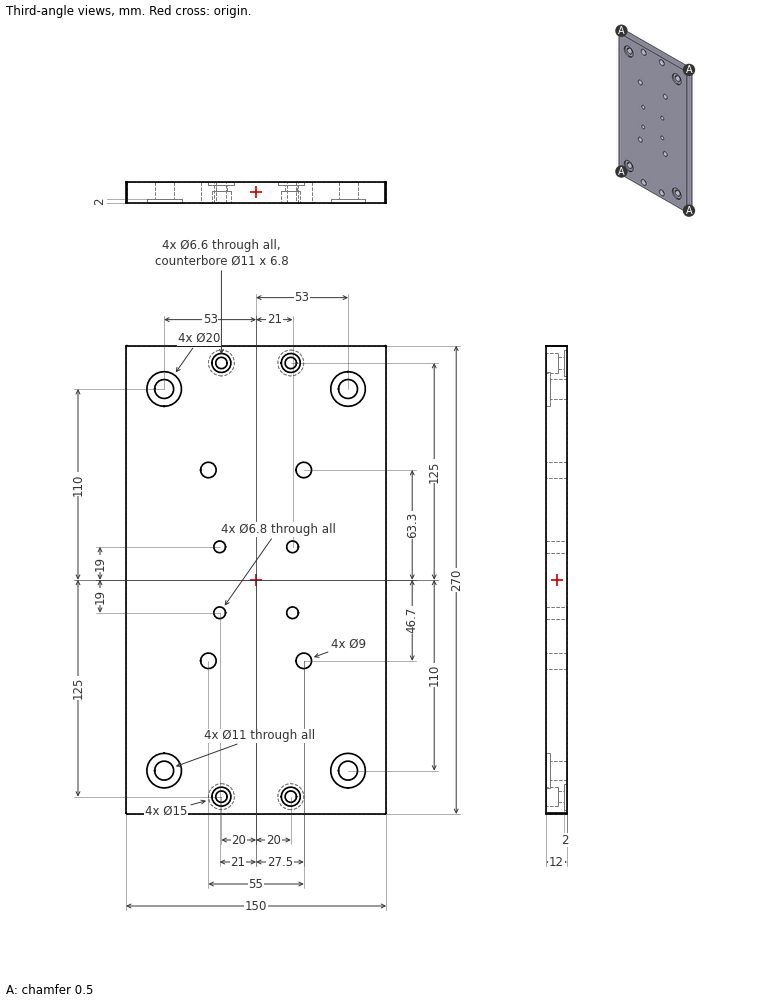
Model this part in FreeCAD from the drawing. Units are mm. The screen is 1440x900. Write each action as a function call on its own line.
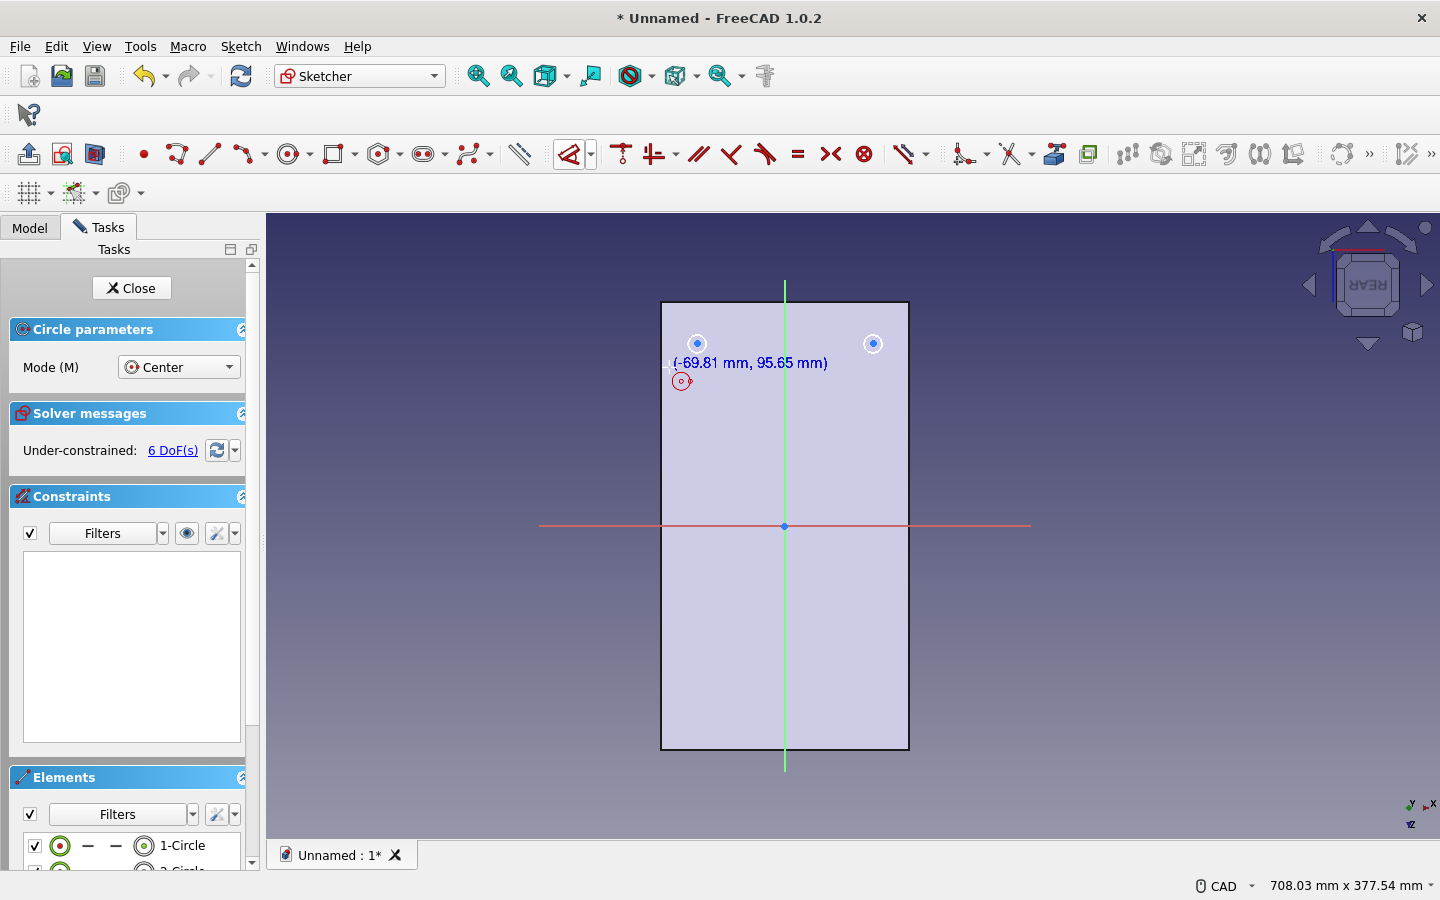
scroll(697, 709, up, 5)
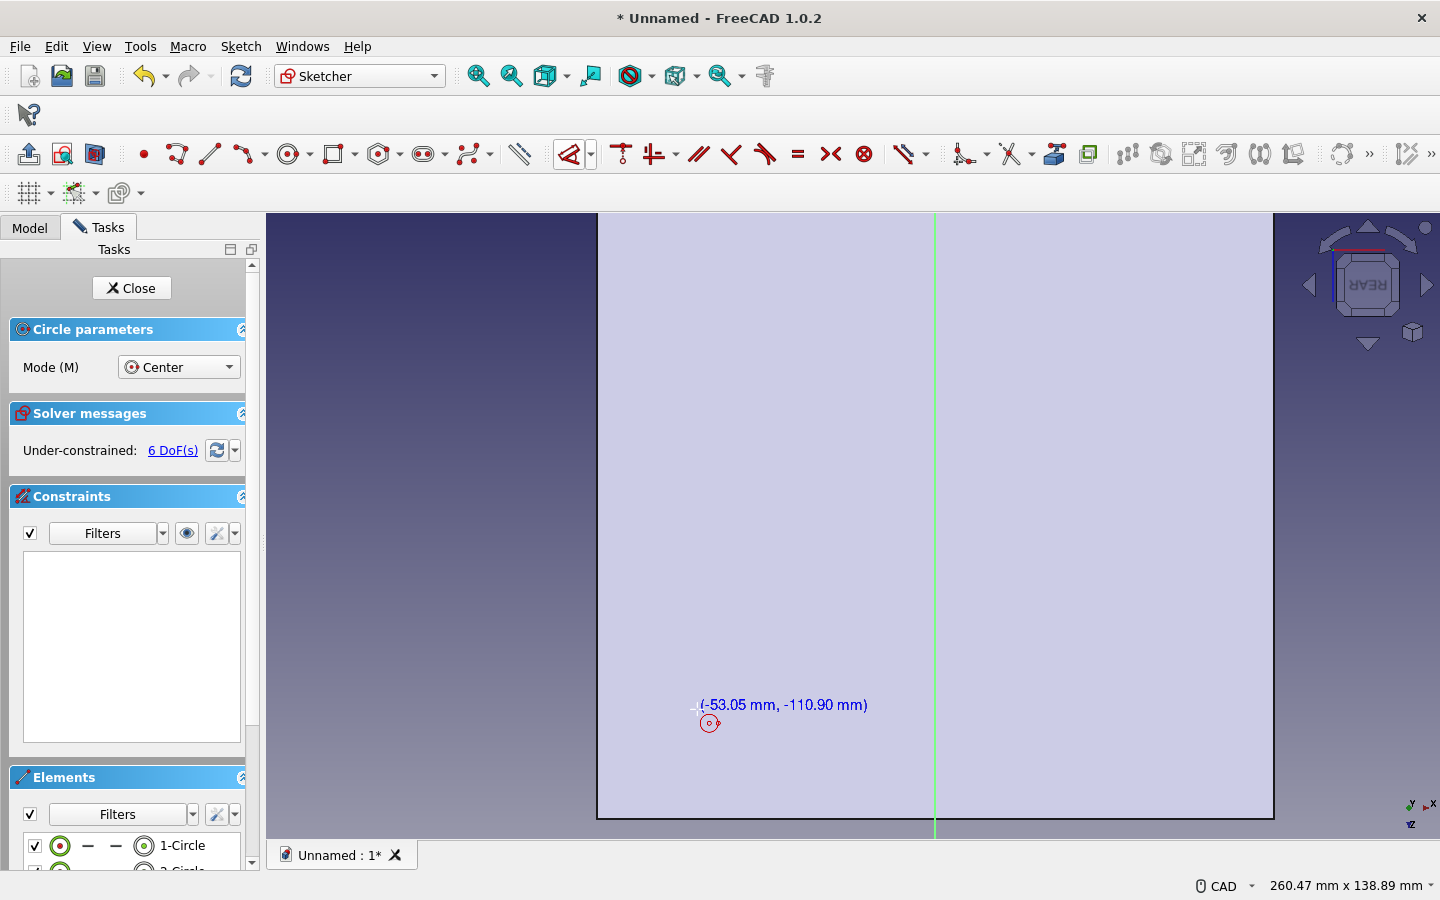
click(697, 706)
click(714, 689)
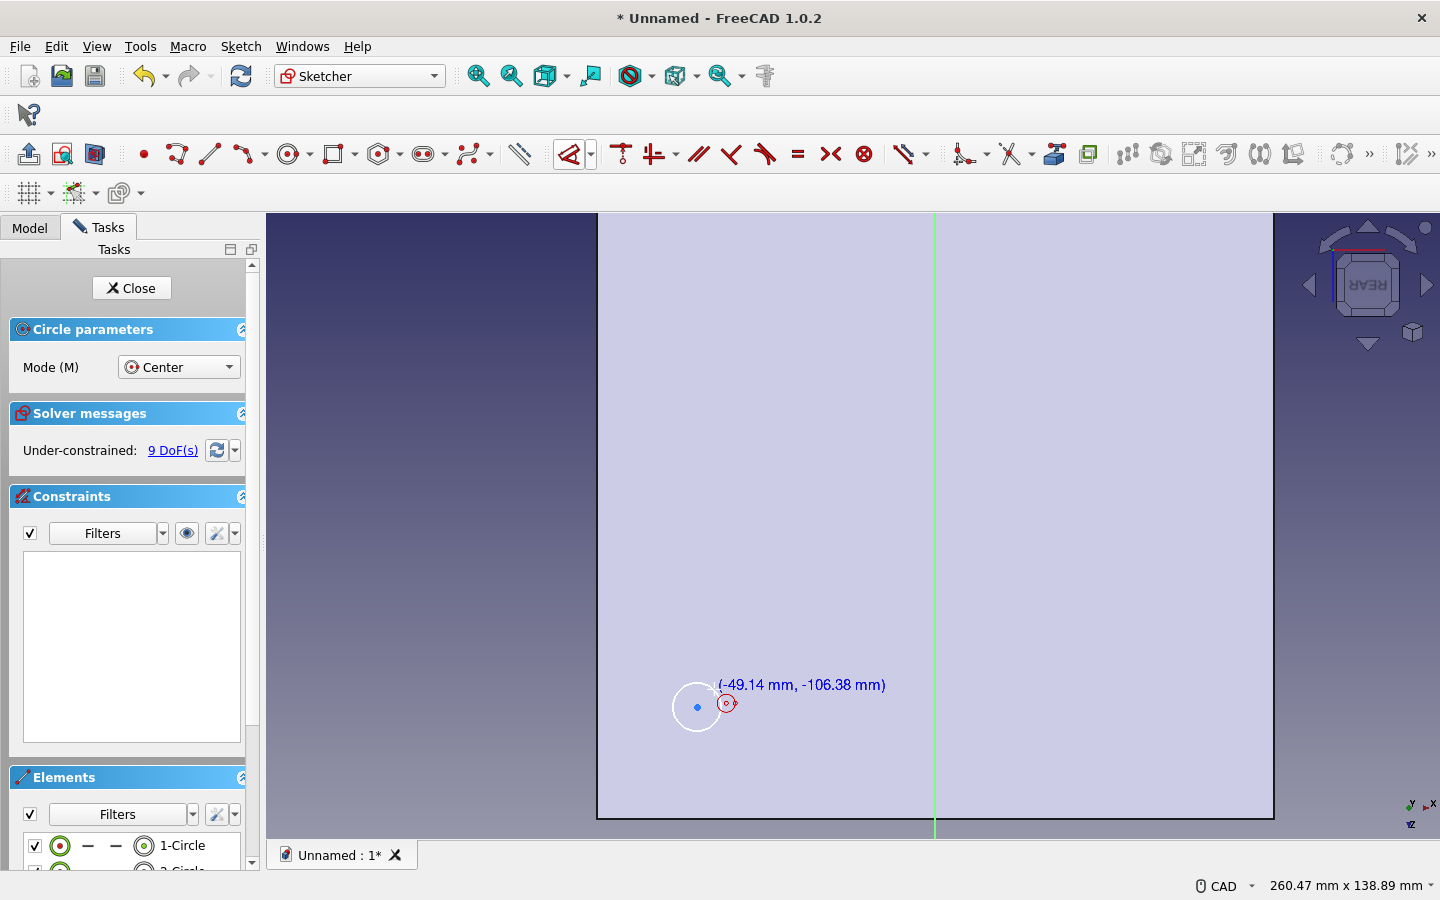
click(1174, 706)
click(1192, 689)
key(Escape)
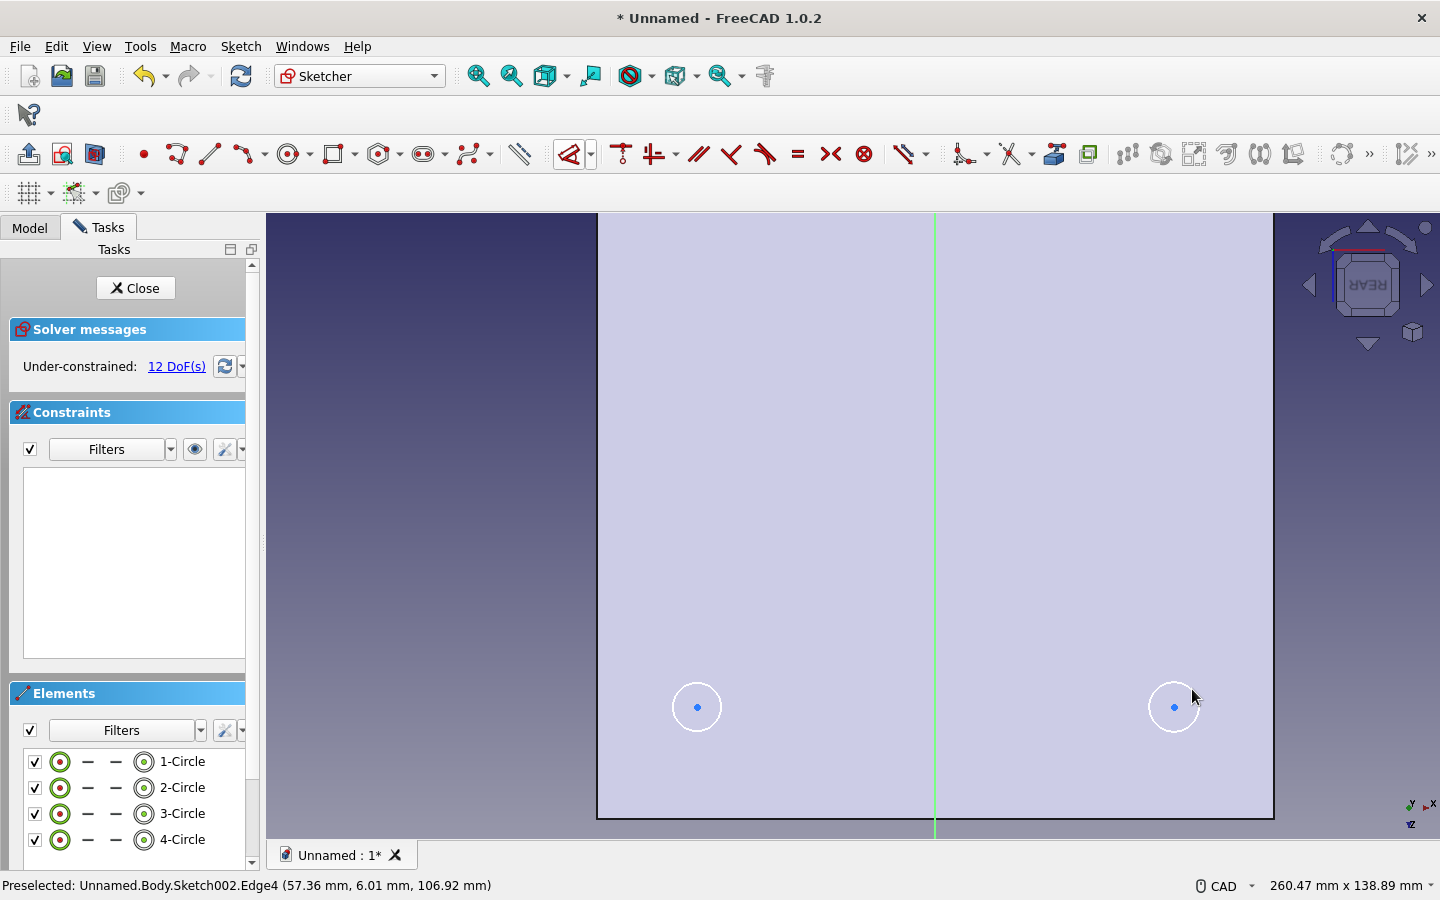
scroll(697, 710, down, 5)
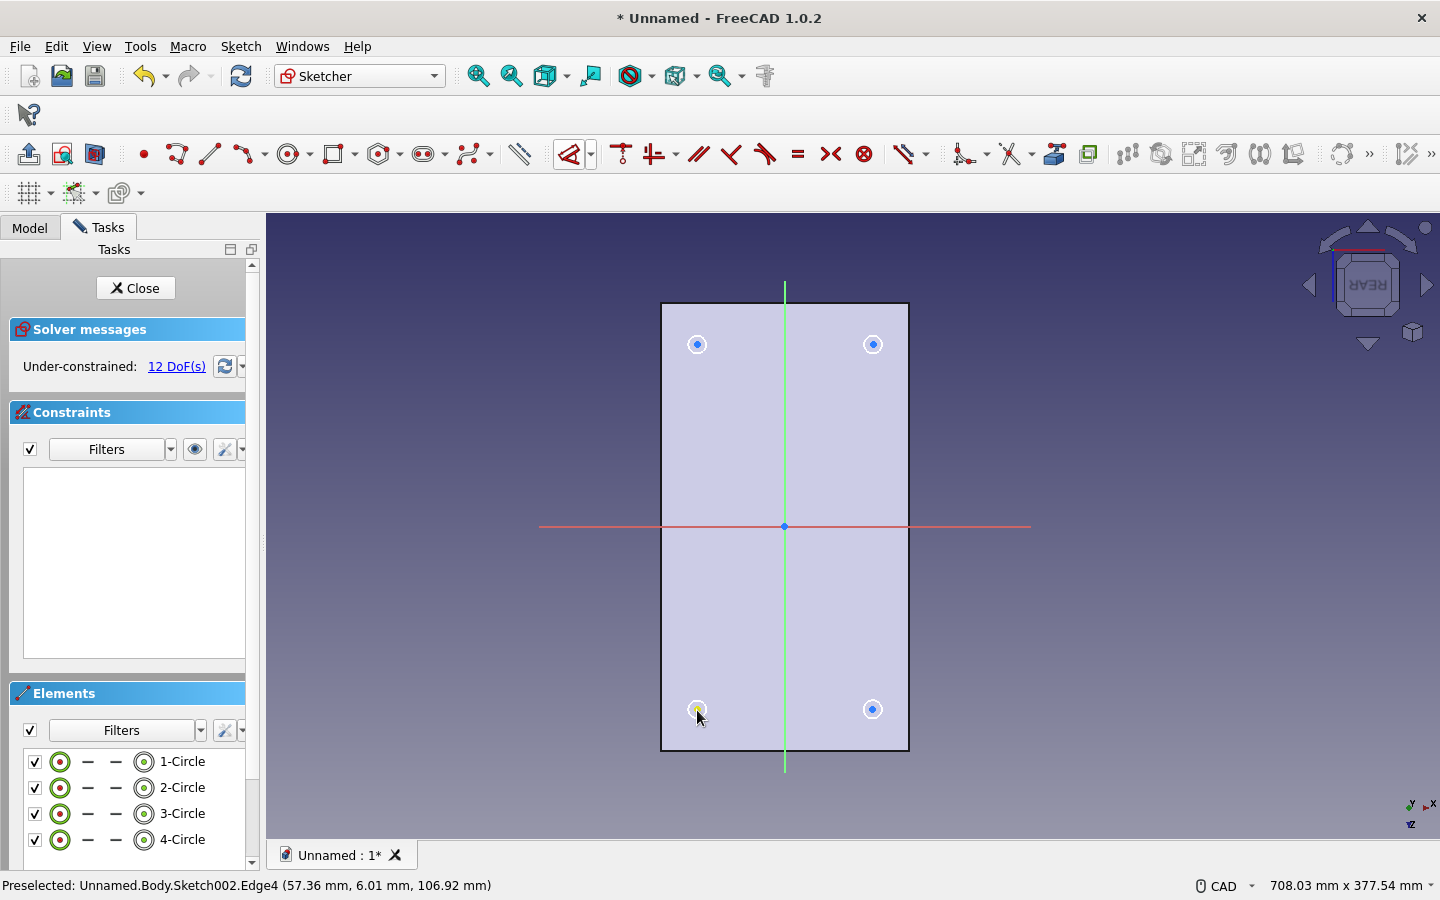
scroll(703, 338, up, 3)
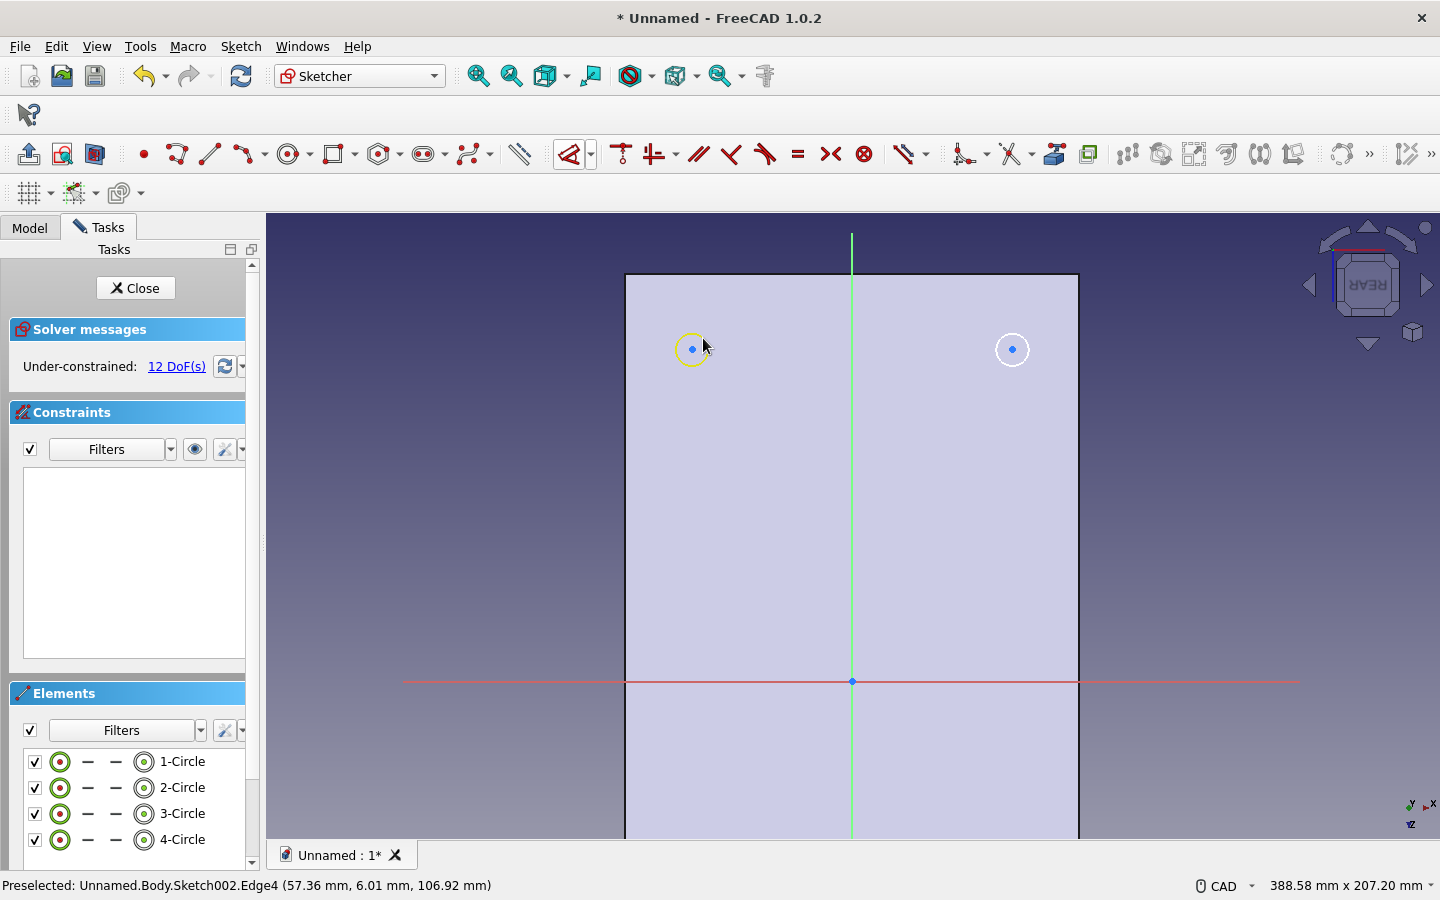
click(703, 338)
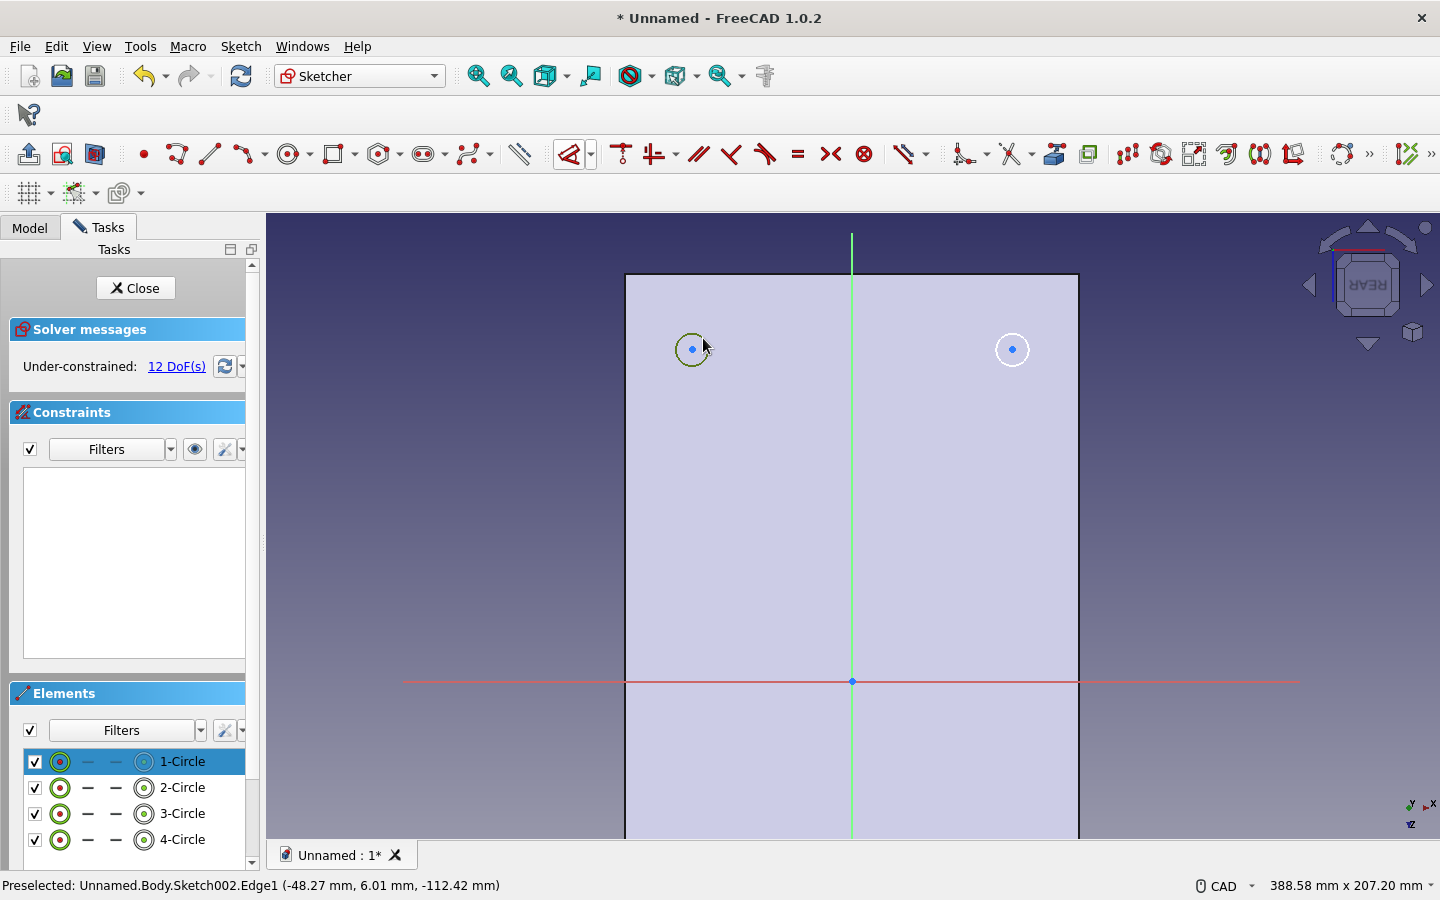
click(1024, 338)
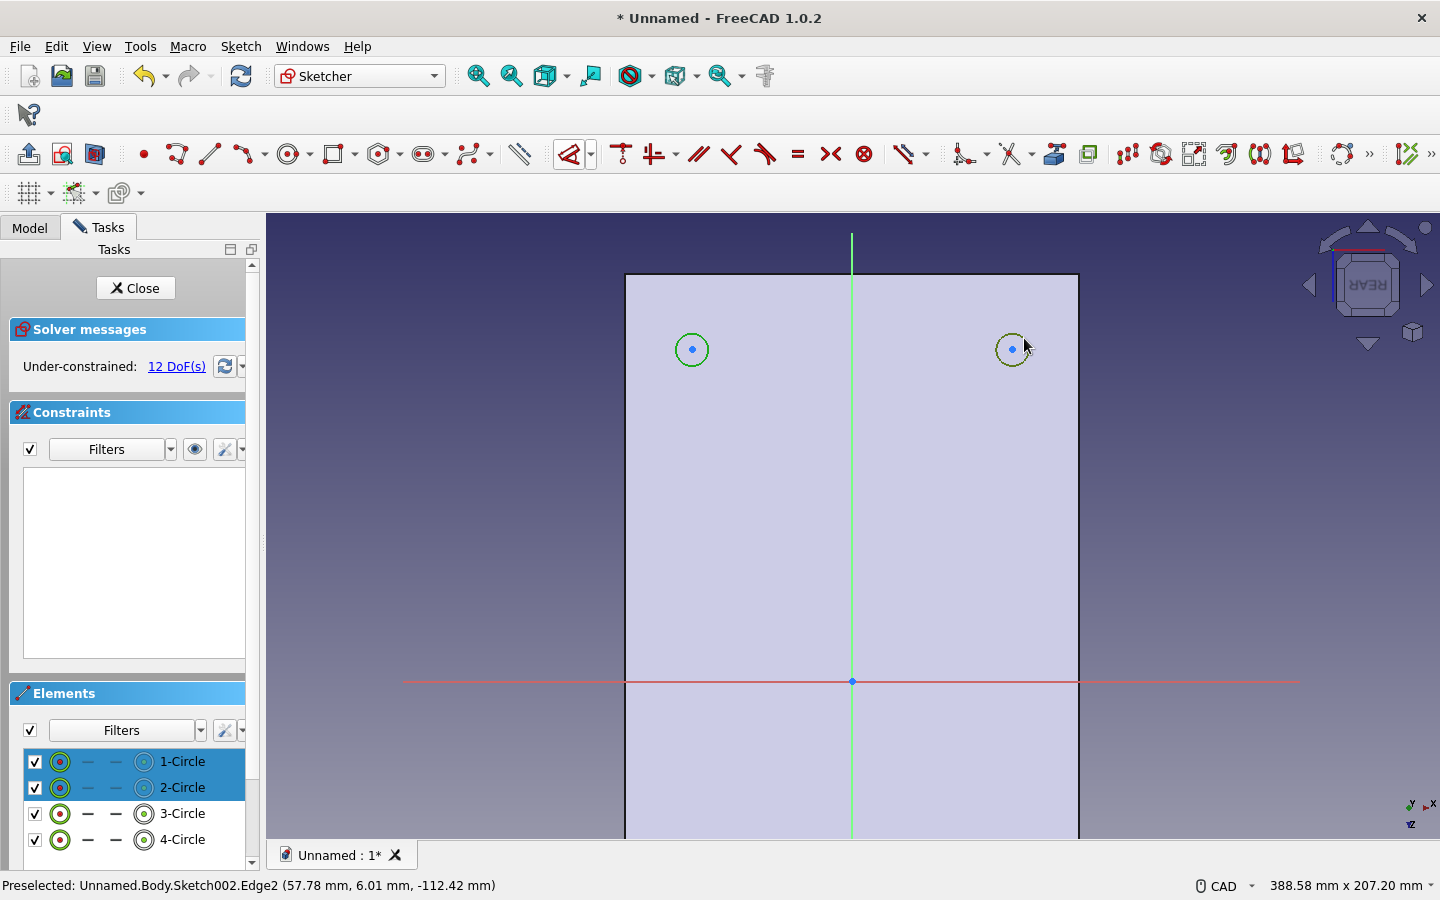
scroll(702, 337, down, 3)